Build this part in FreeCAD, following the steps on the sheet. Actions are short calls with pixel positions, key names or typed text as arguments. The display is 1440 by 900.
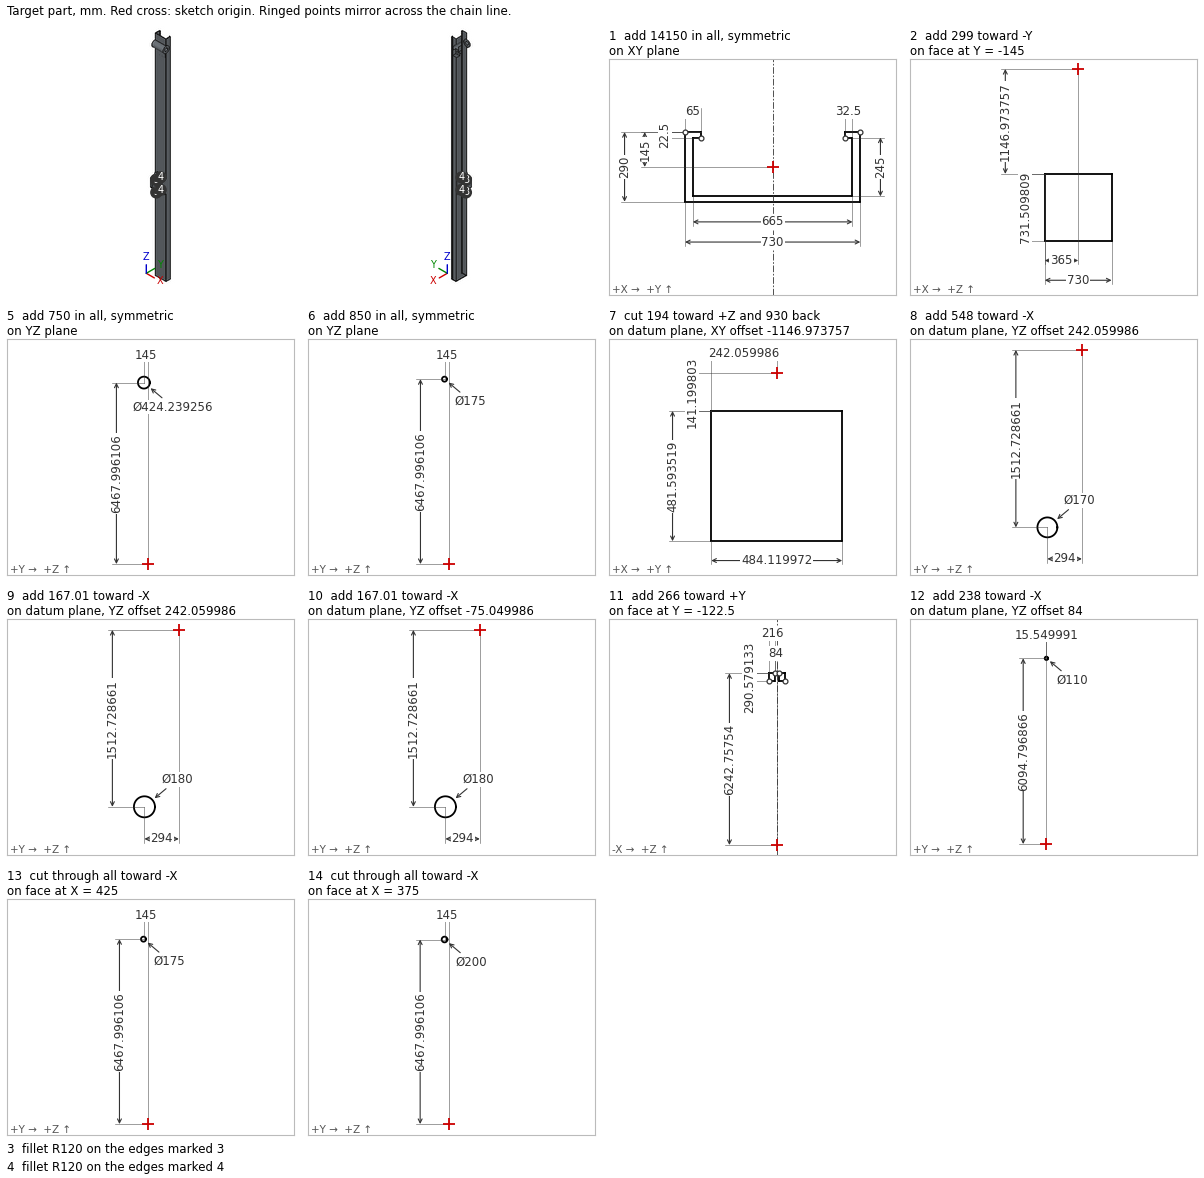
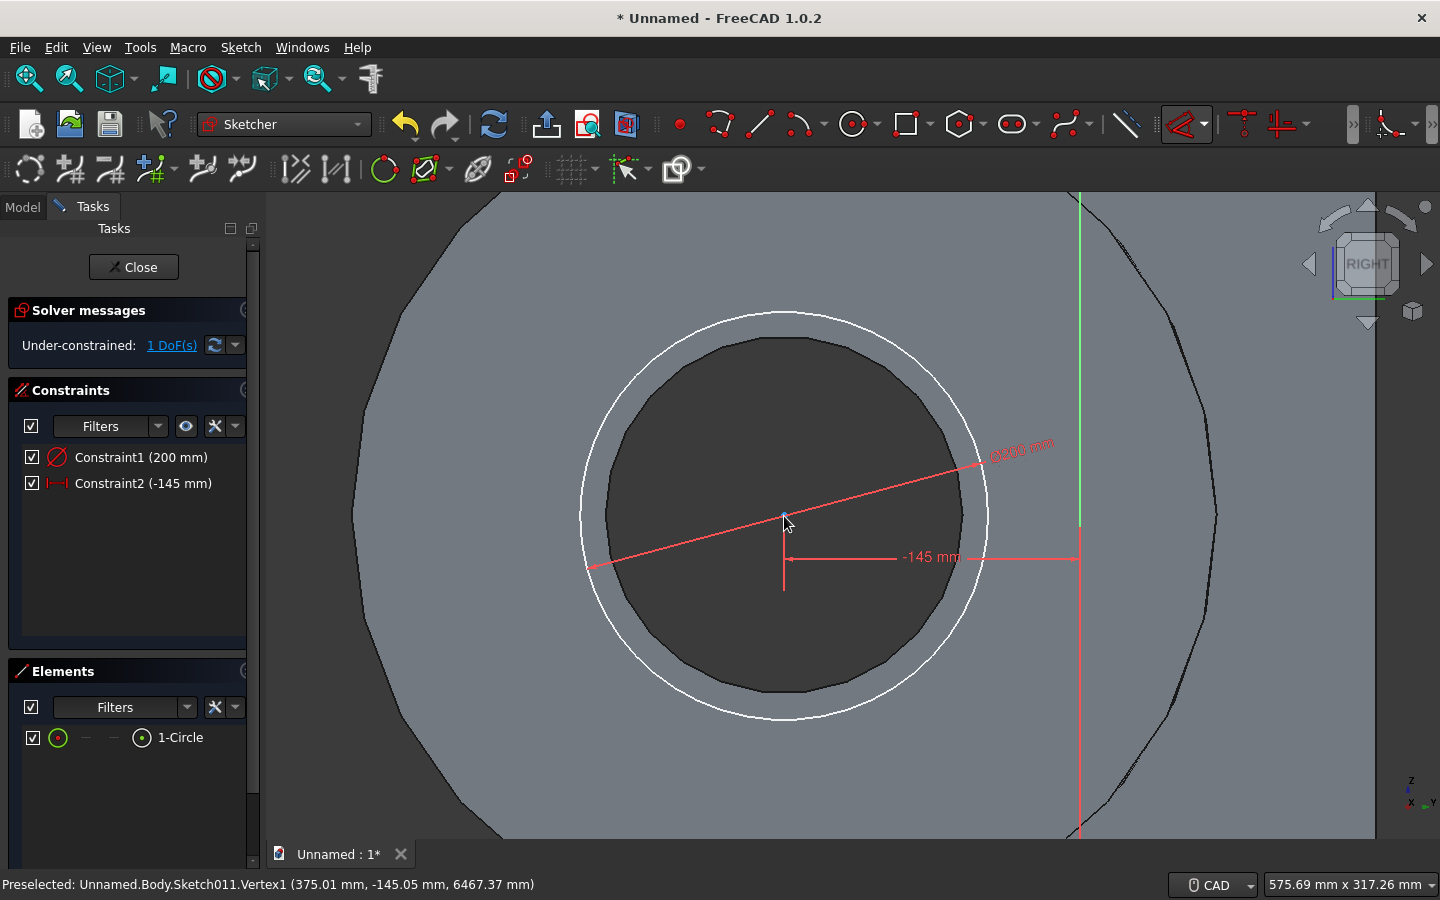
click(784, 516)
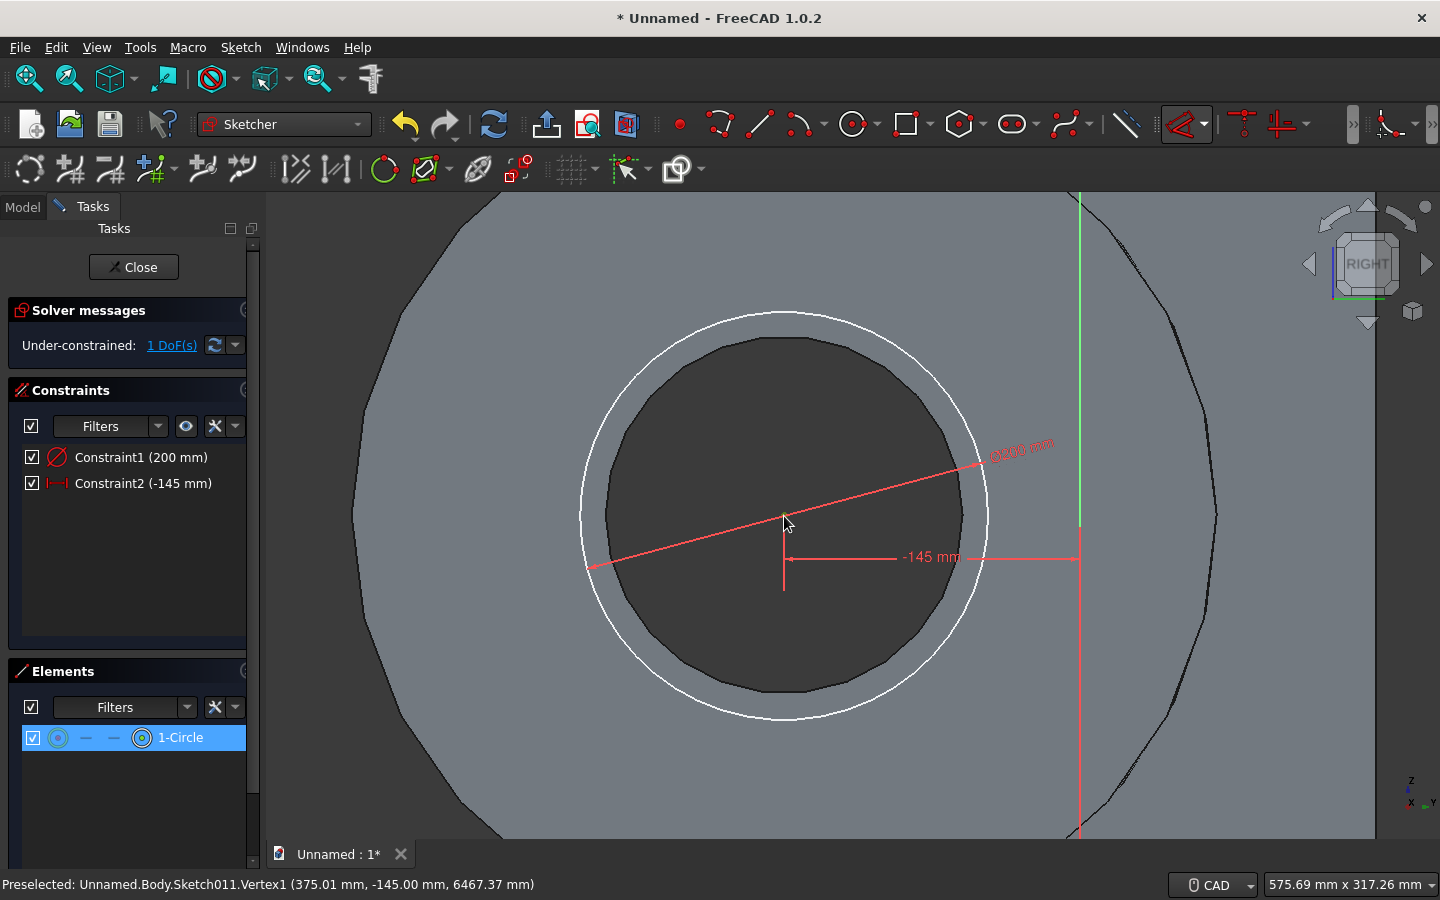
key(i)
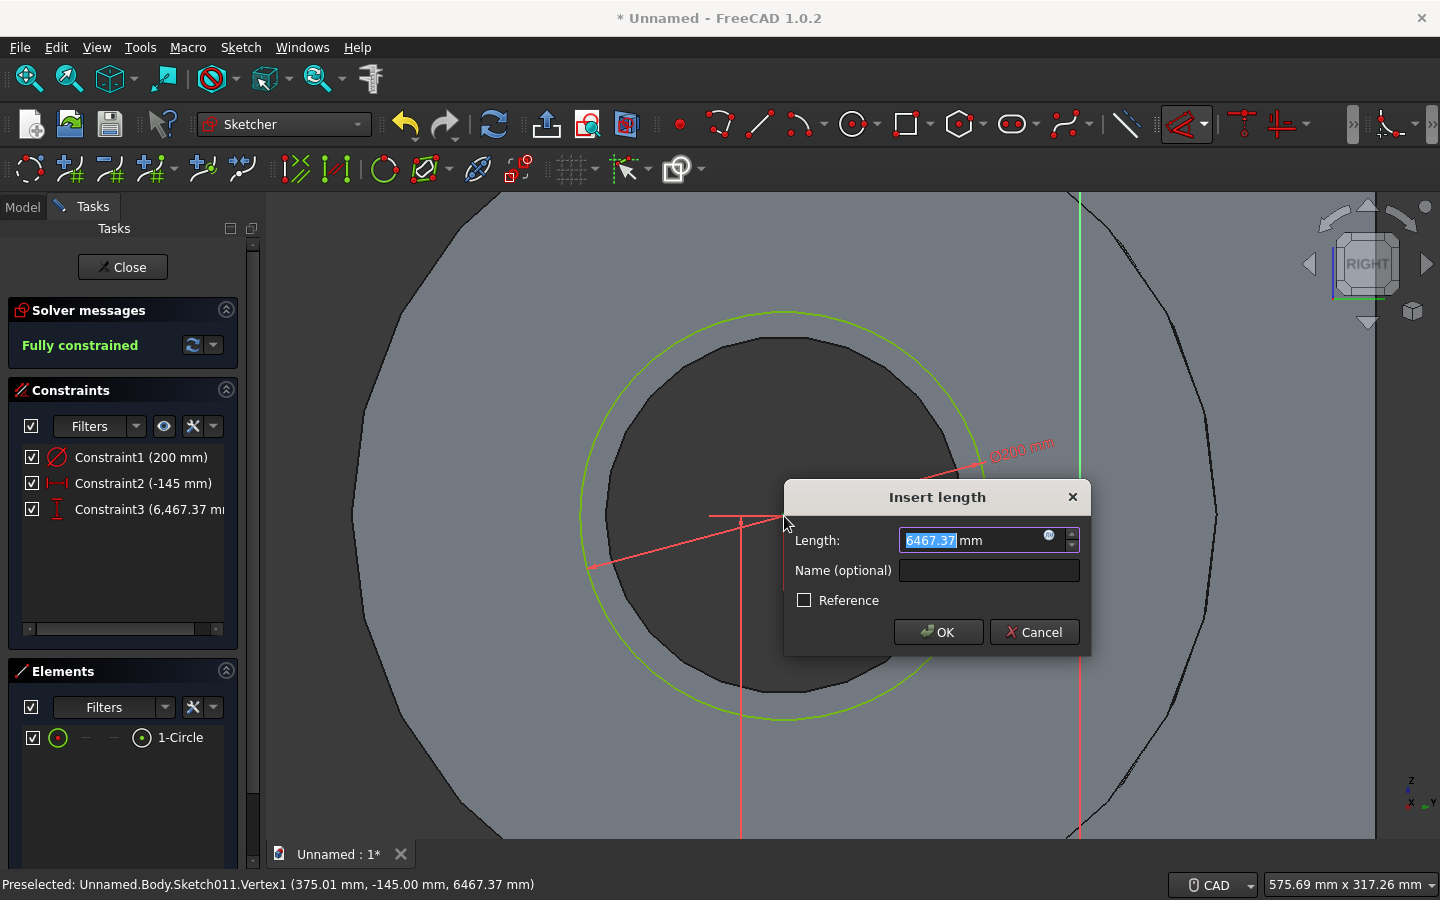
text(6467.996106)
key(Return)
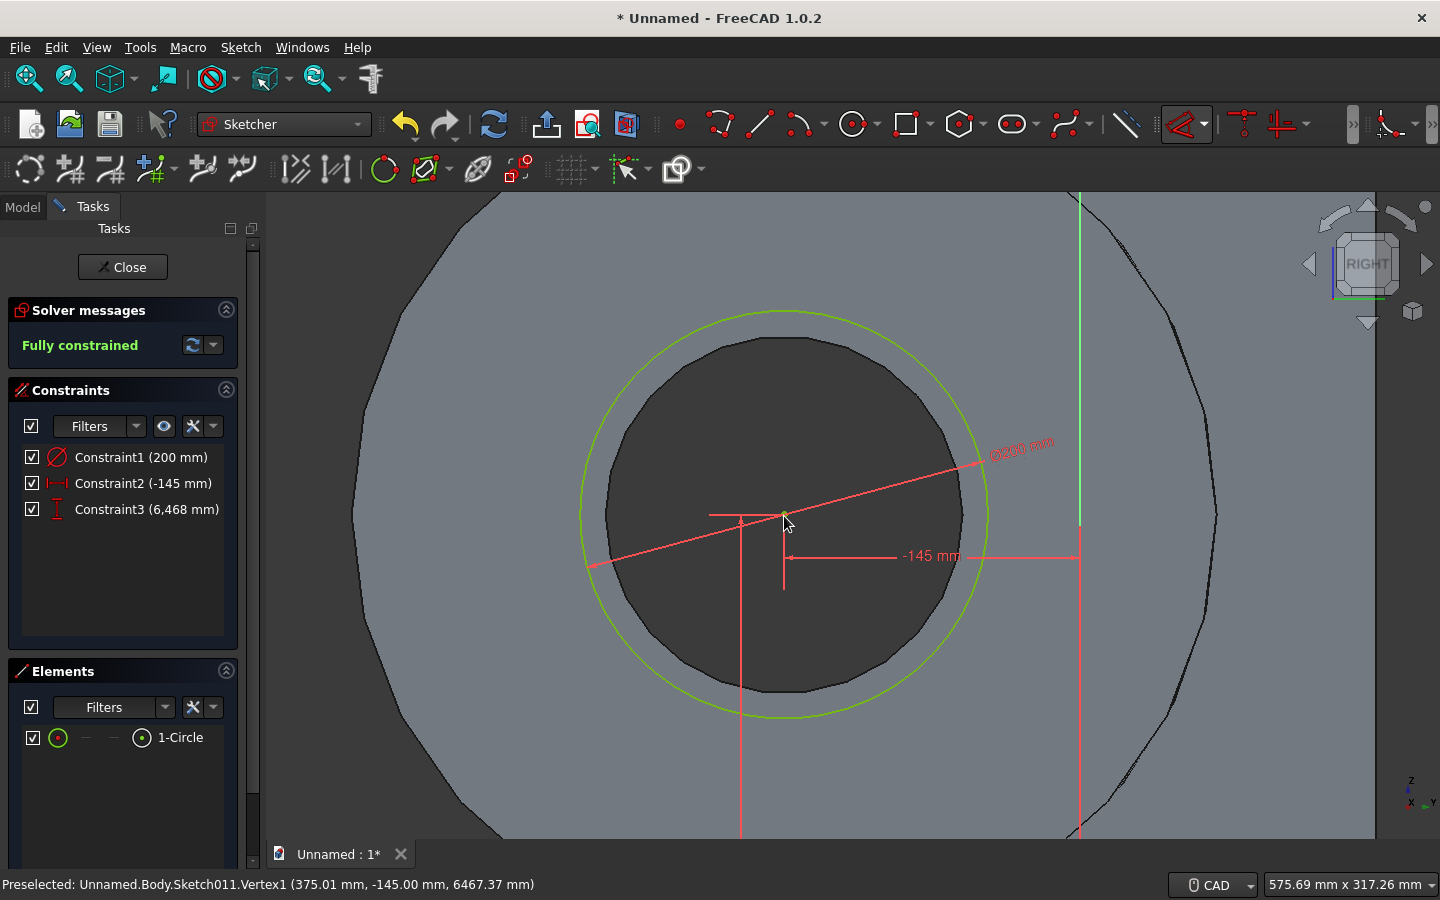
click(123, 267)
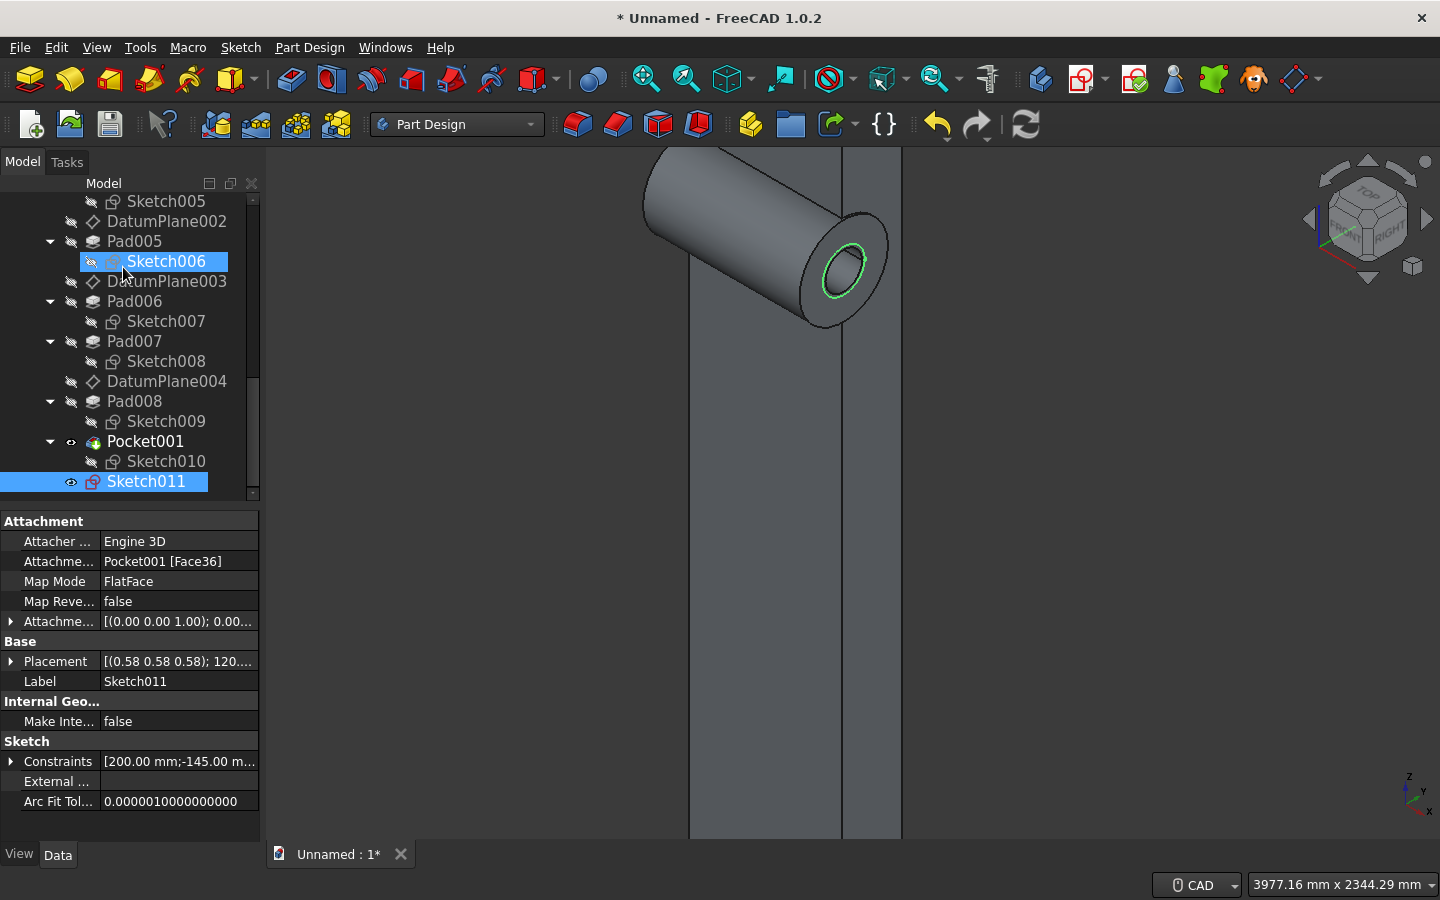
click(292, 80)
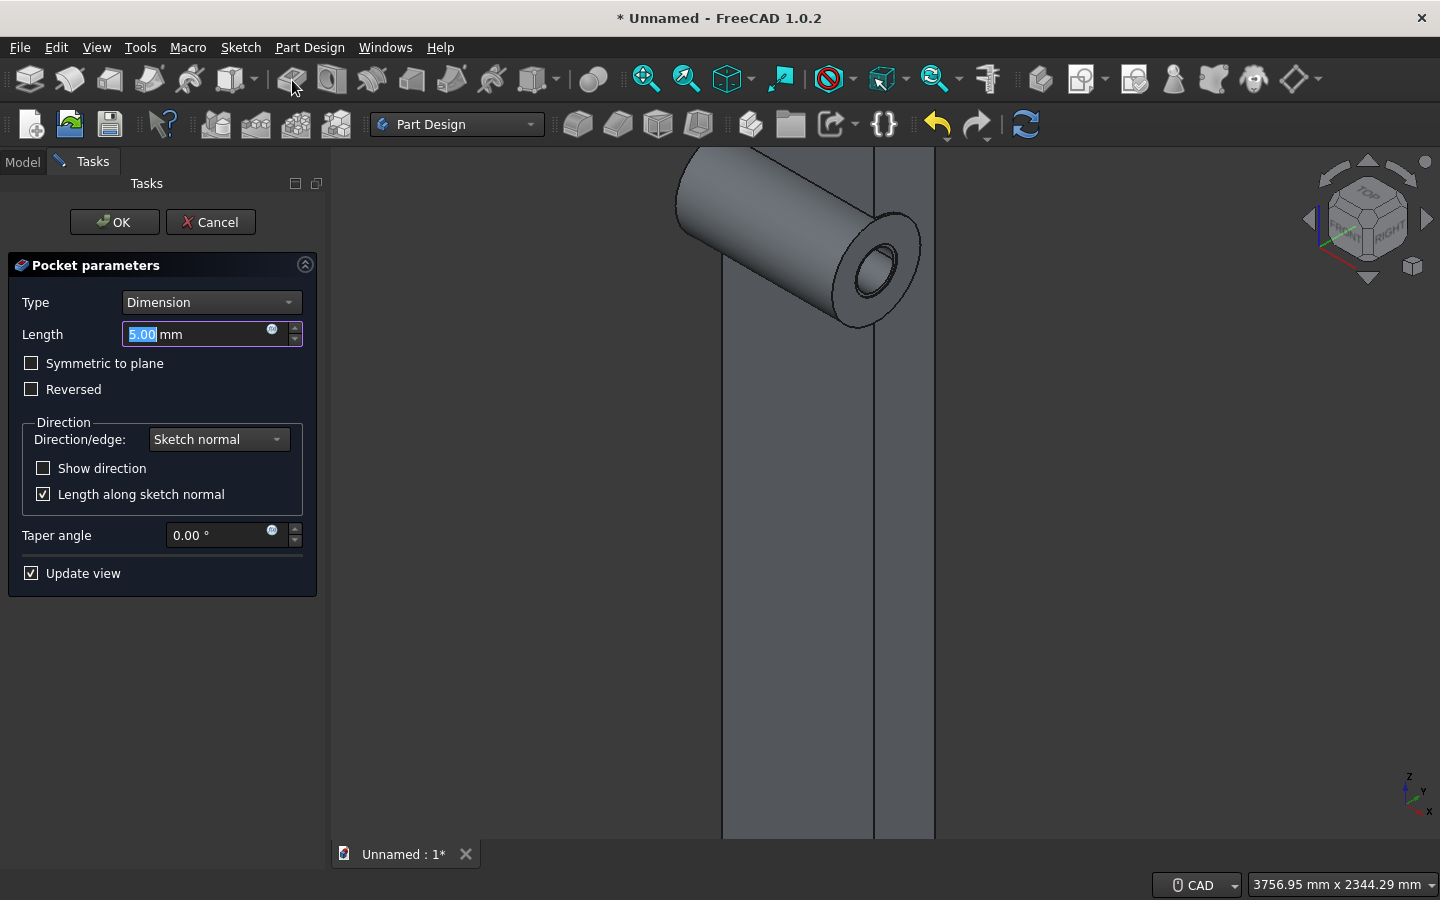
click(212, 302)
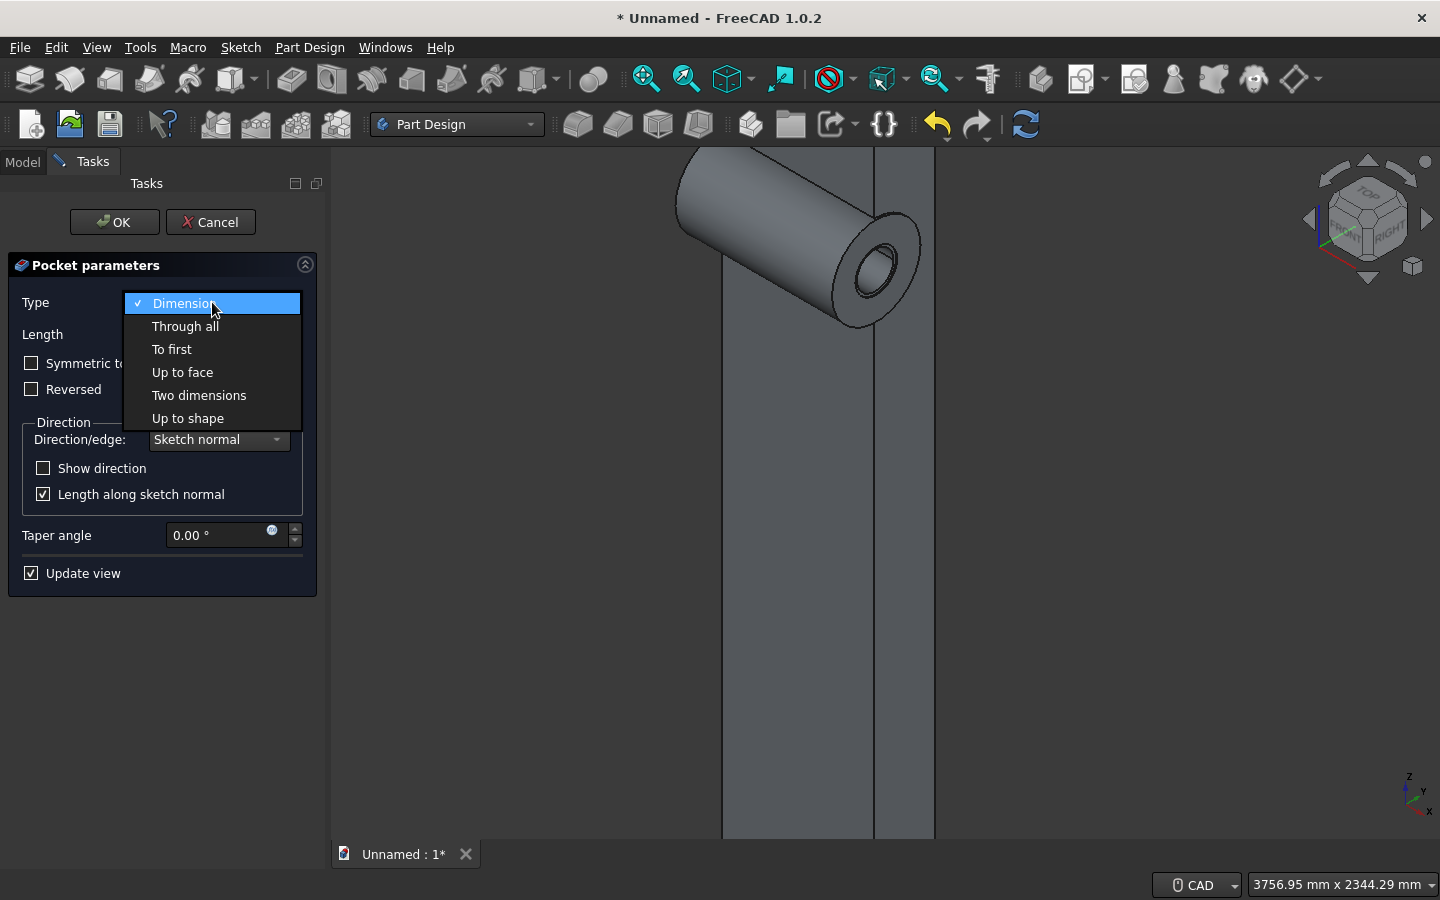
click(212, 326)